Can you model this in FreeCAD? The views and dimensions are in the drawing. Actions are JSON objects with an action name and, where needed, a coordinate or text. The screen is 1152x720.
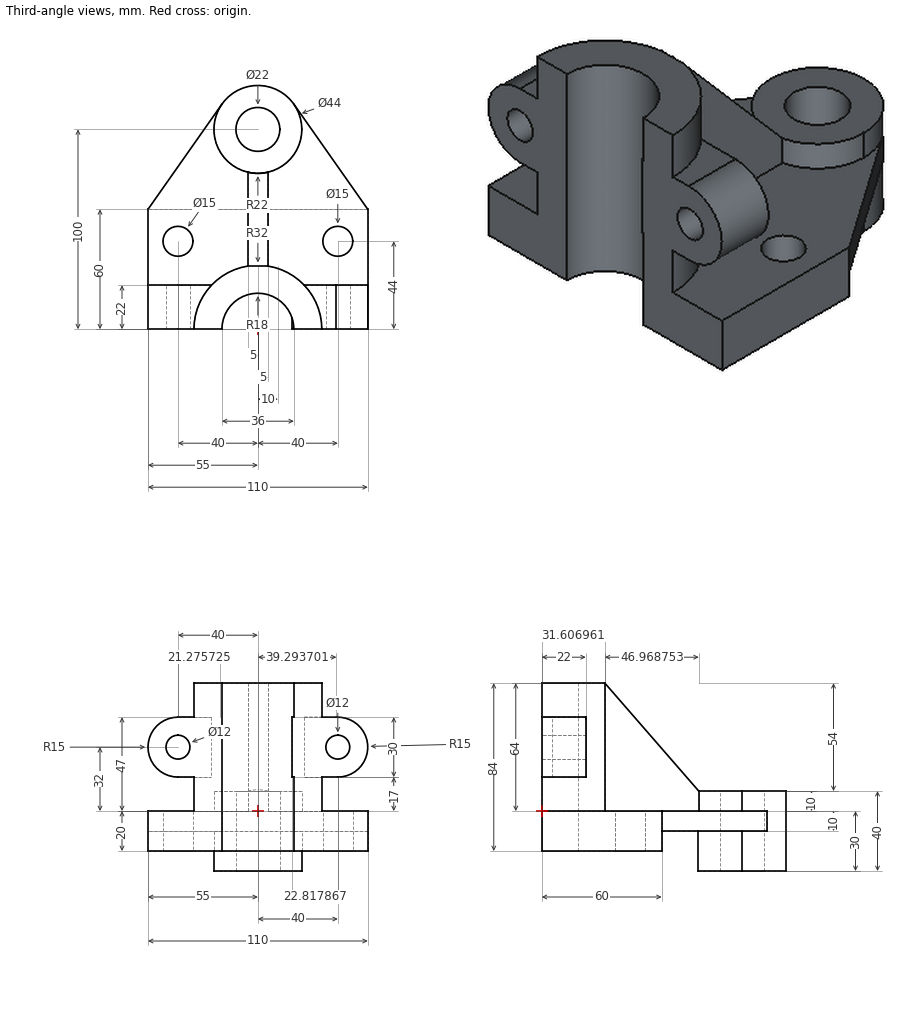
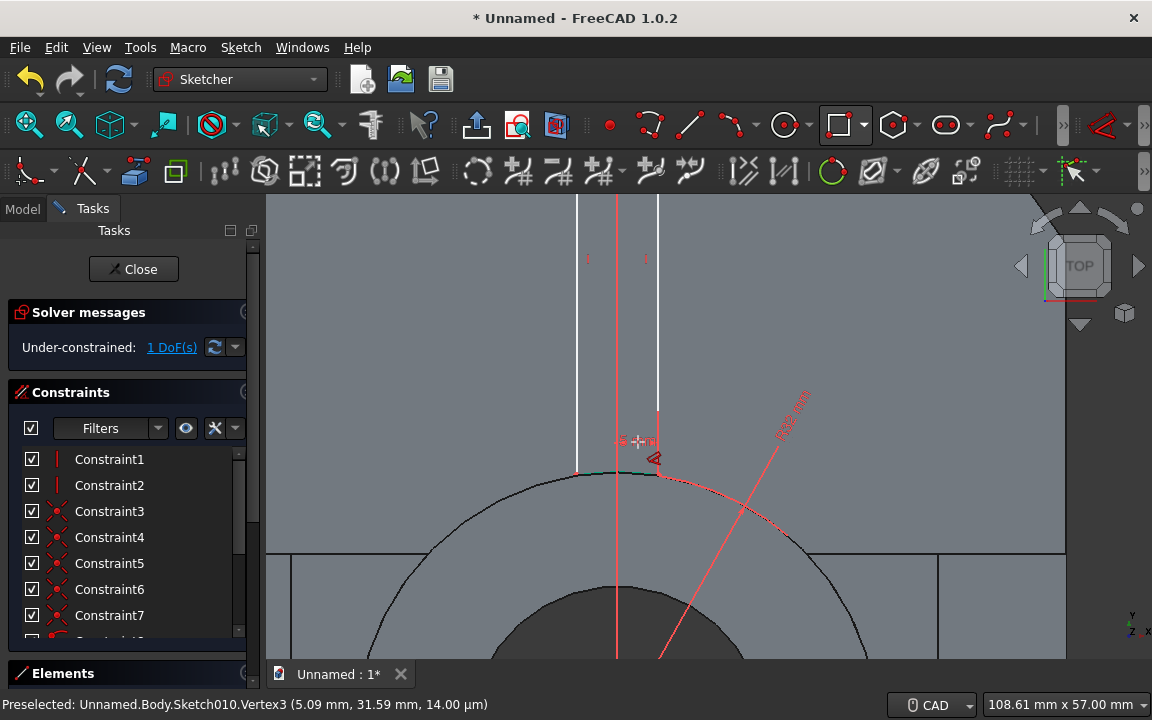
{"action": "scroll", "coordinate": [659, 438], "scroll_direction": "down", "scroll_amount": 4}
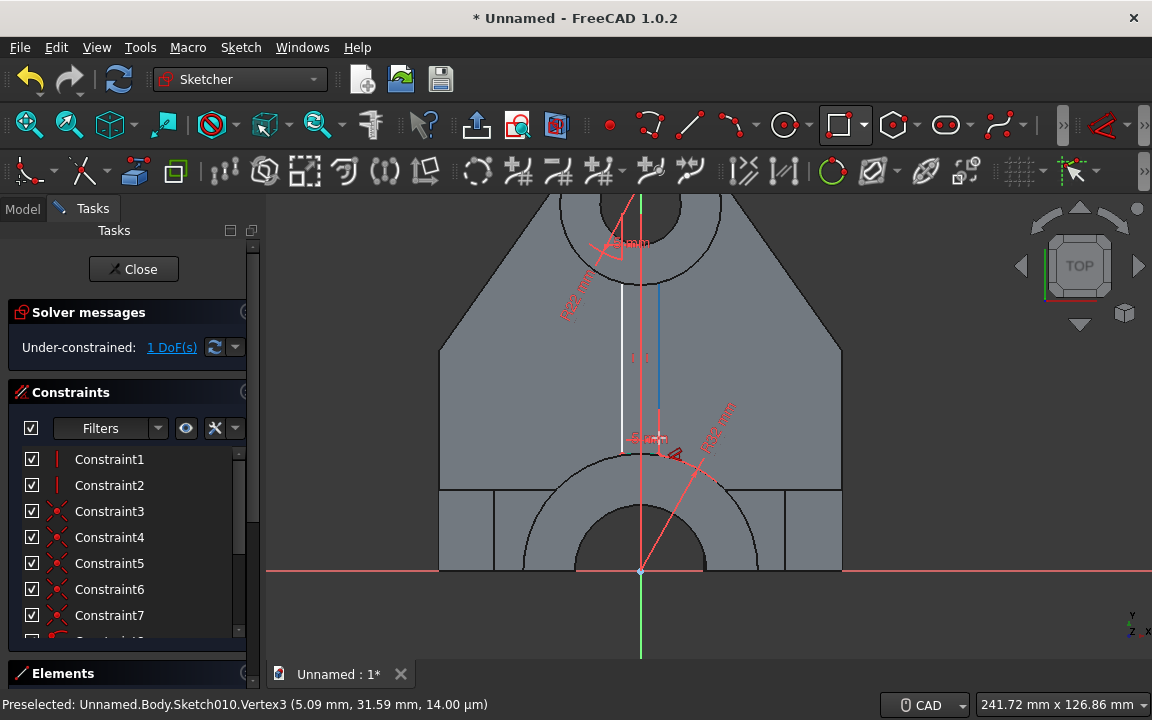
{"action": "scroll", "coordinate": [640, 631], "scroll_direction": "down", "scroll_amount": 1}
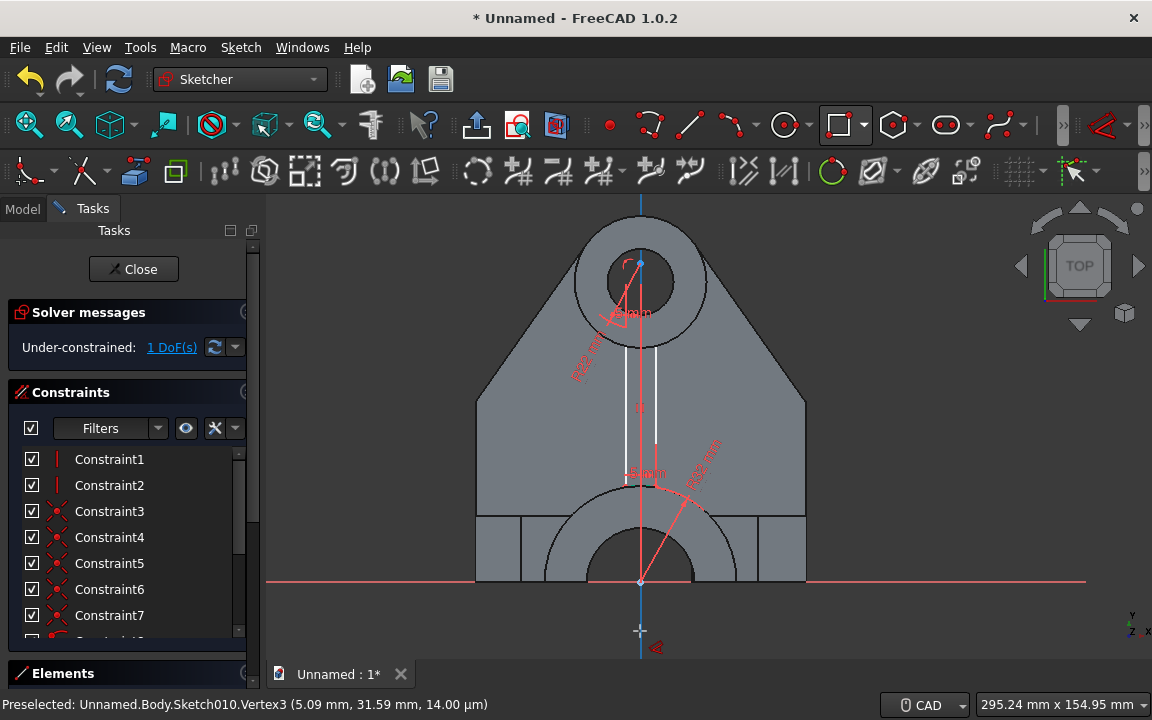
{"action": "left_click", "coordinate": [641, 263]}
{"action": "left_click", "coordinate": [675, 423]}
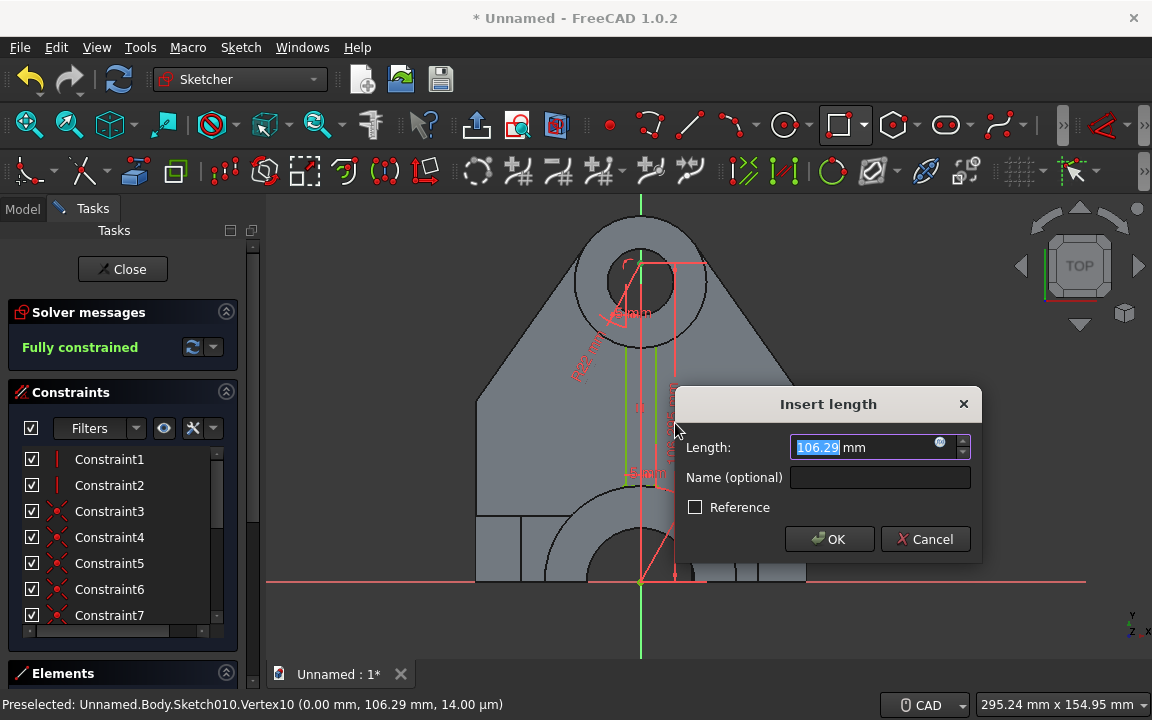
{"action": "type", "text": "100"}
{"action": "key", "text": "Return"}
{"action": "key", "text": "Escape"}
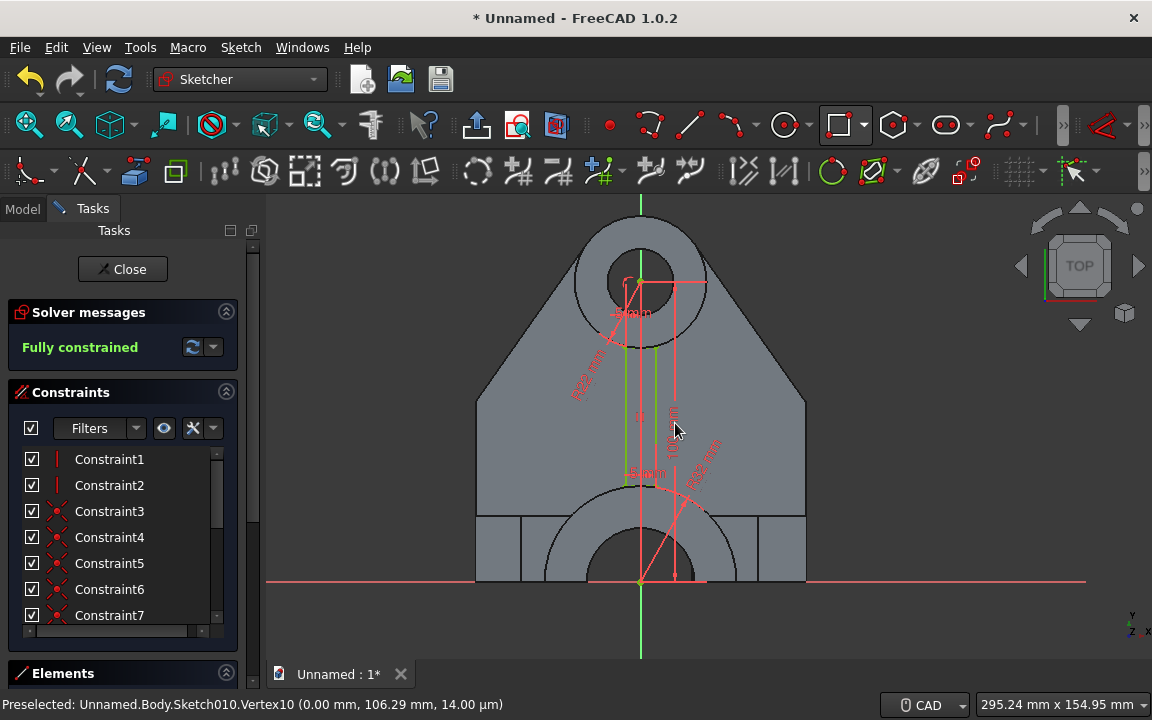
{"action": "left_click", "coordinate": [123, 269]}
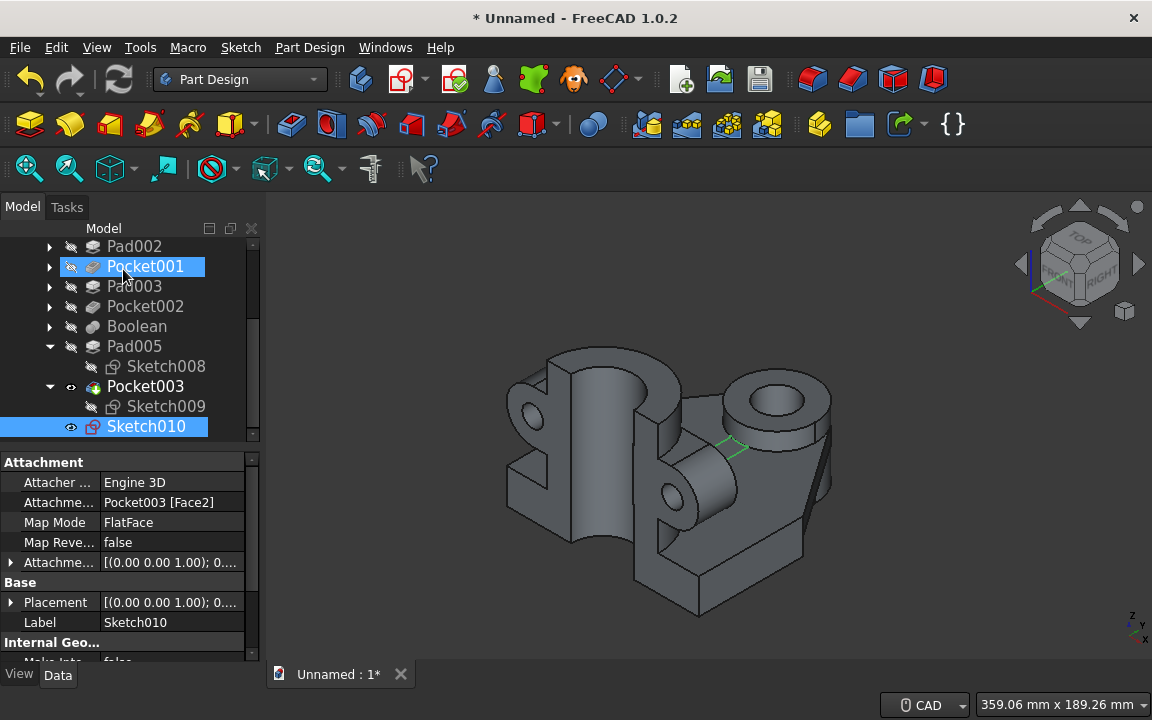
{"action": "left_click", "coordinate": [30, 124]}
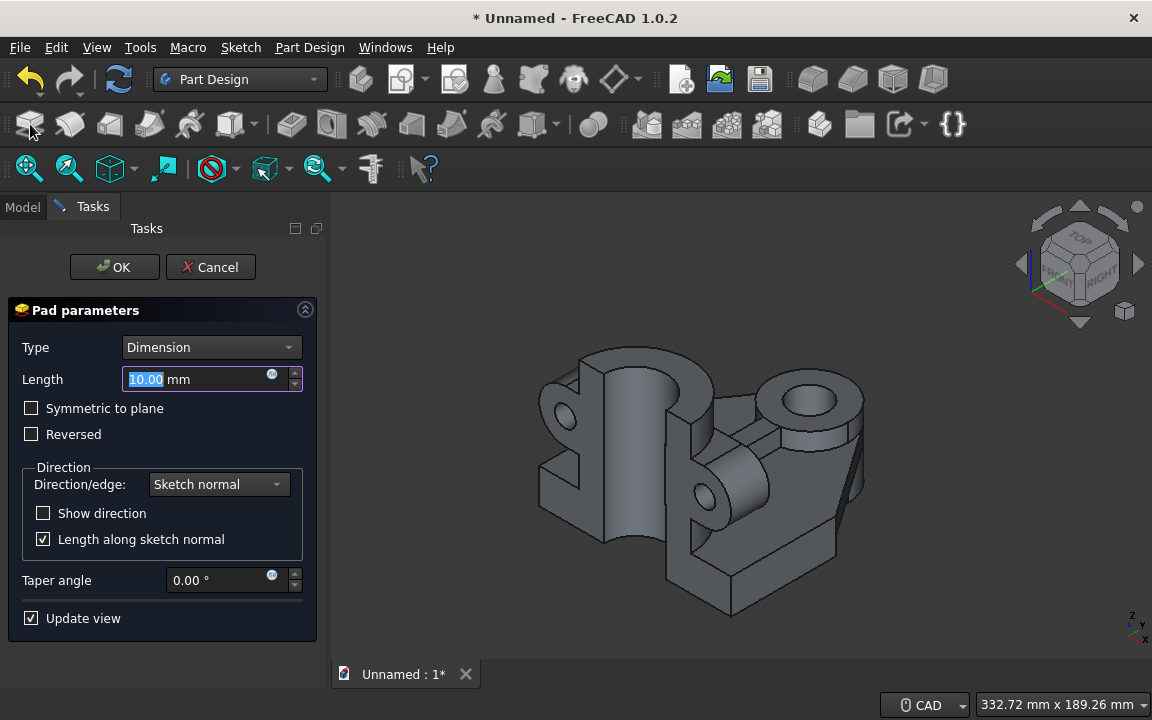
{"action": "type", "text": "64"}
{"action": "key", "text": "Tab"}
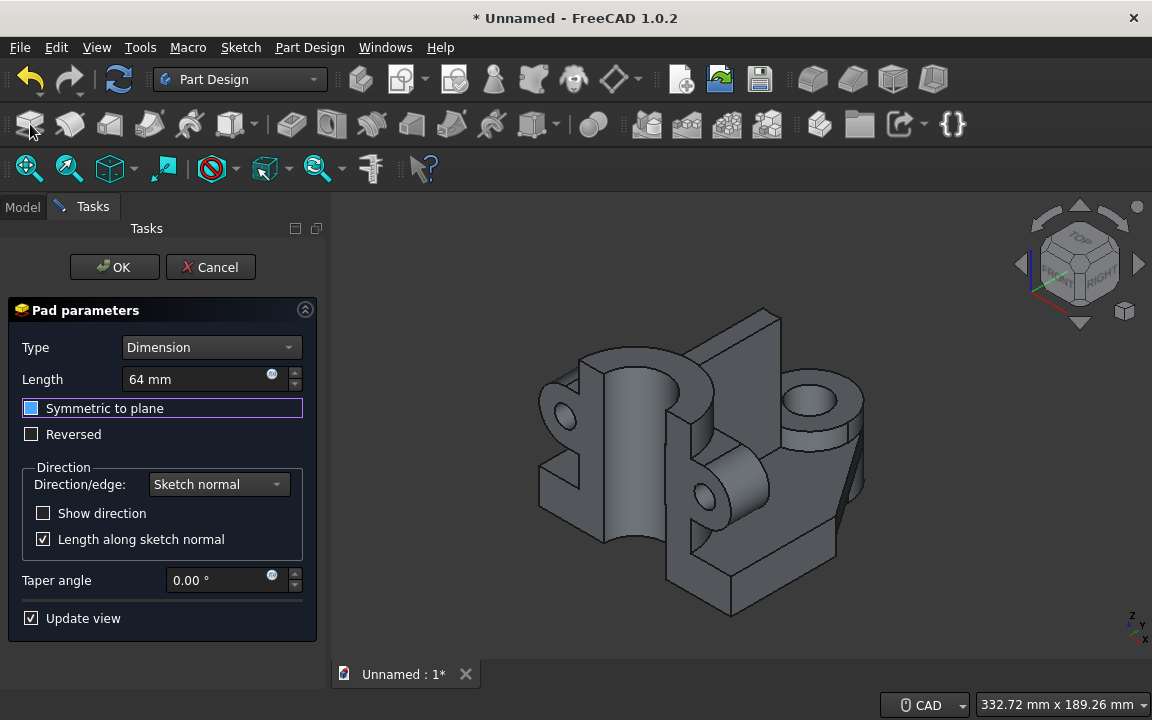
{"action": "left_click", "coordinate": [115, 267]}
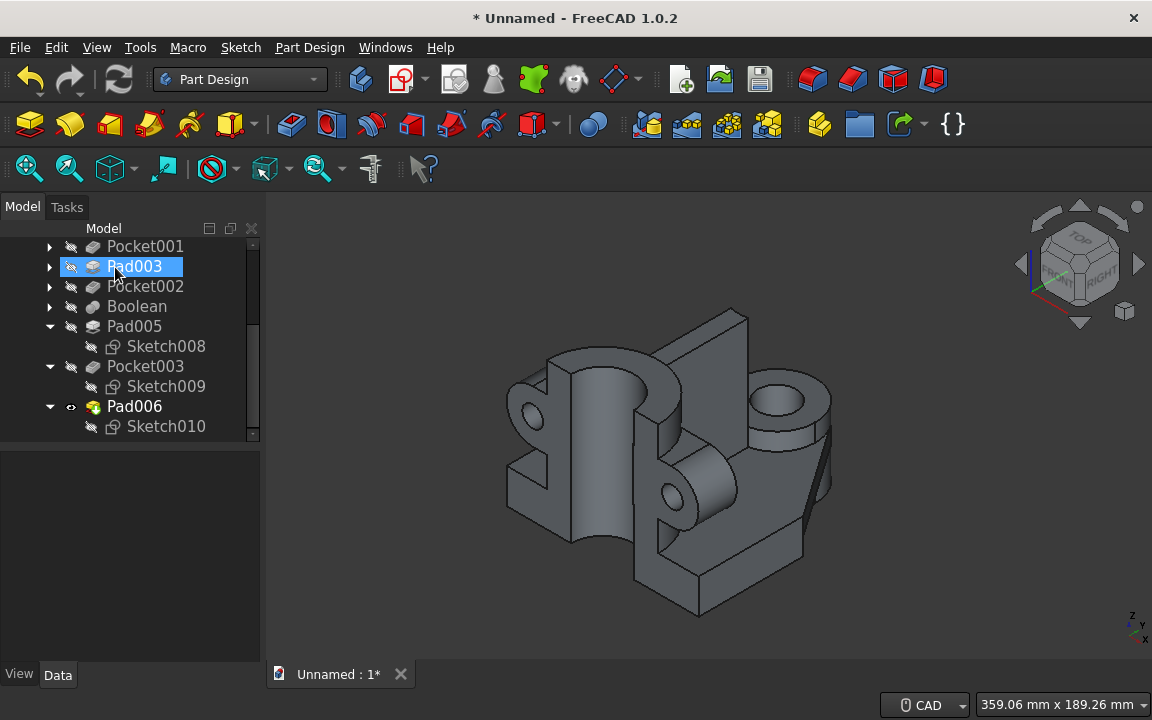
{"action": "left_click", "coordinate": [402, 80]}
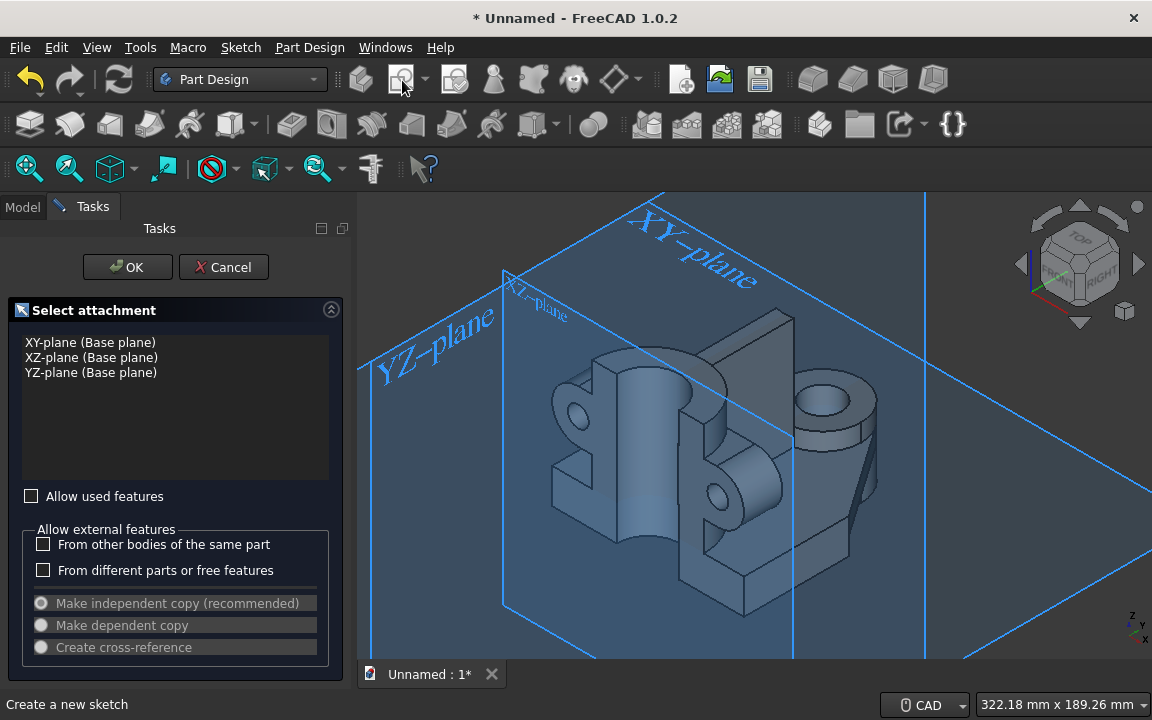
{"action": "left_click", "coordinate": [82, 372]}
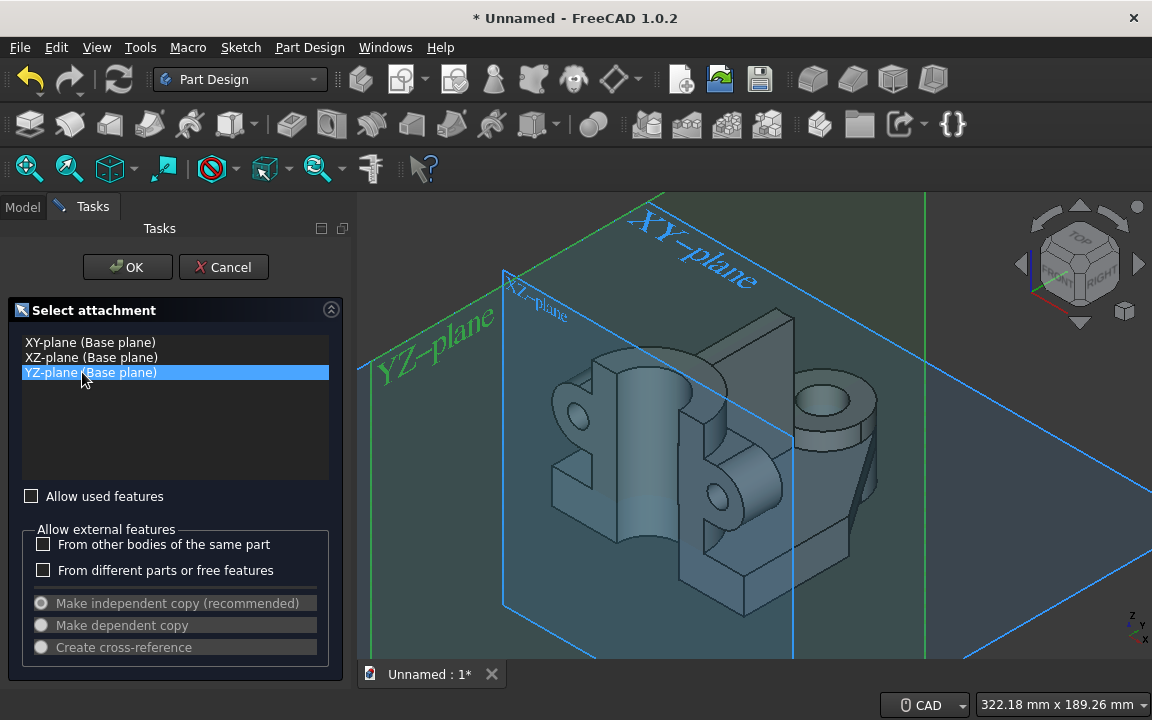
{"action": "left_click", "coordinate": [128, 267]}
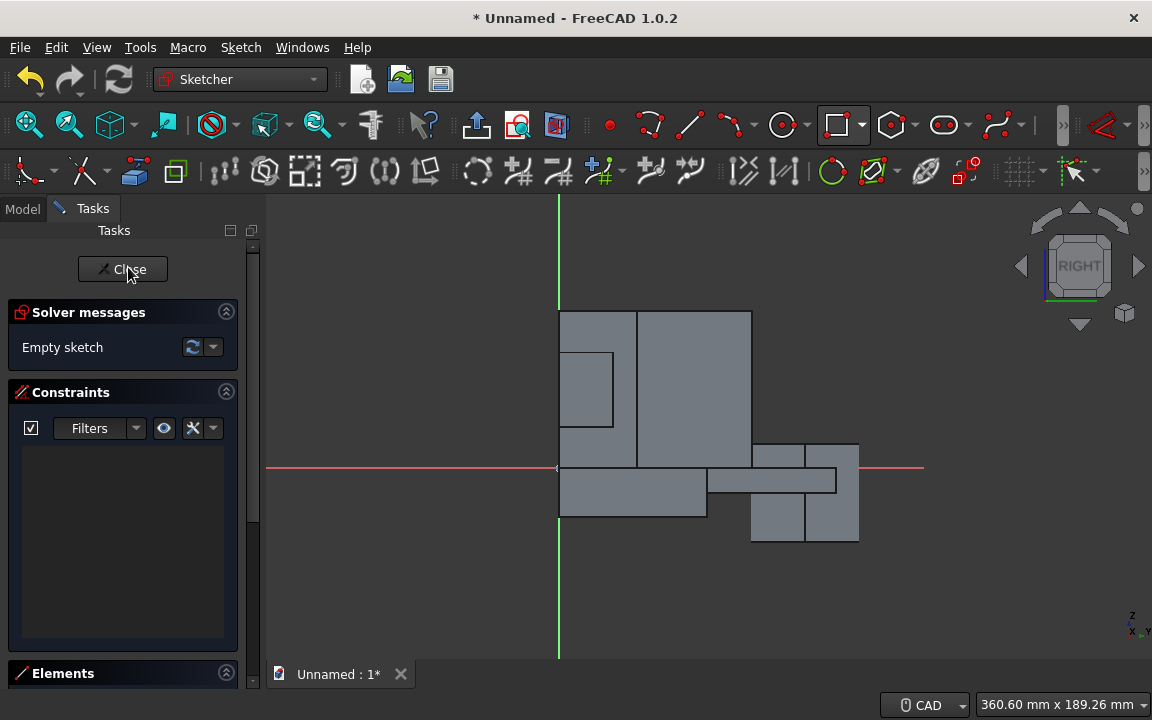
{"action": "left_click", "coordinate": [558, 126]}